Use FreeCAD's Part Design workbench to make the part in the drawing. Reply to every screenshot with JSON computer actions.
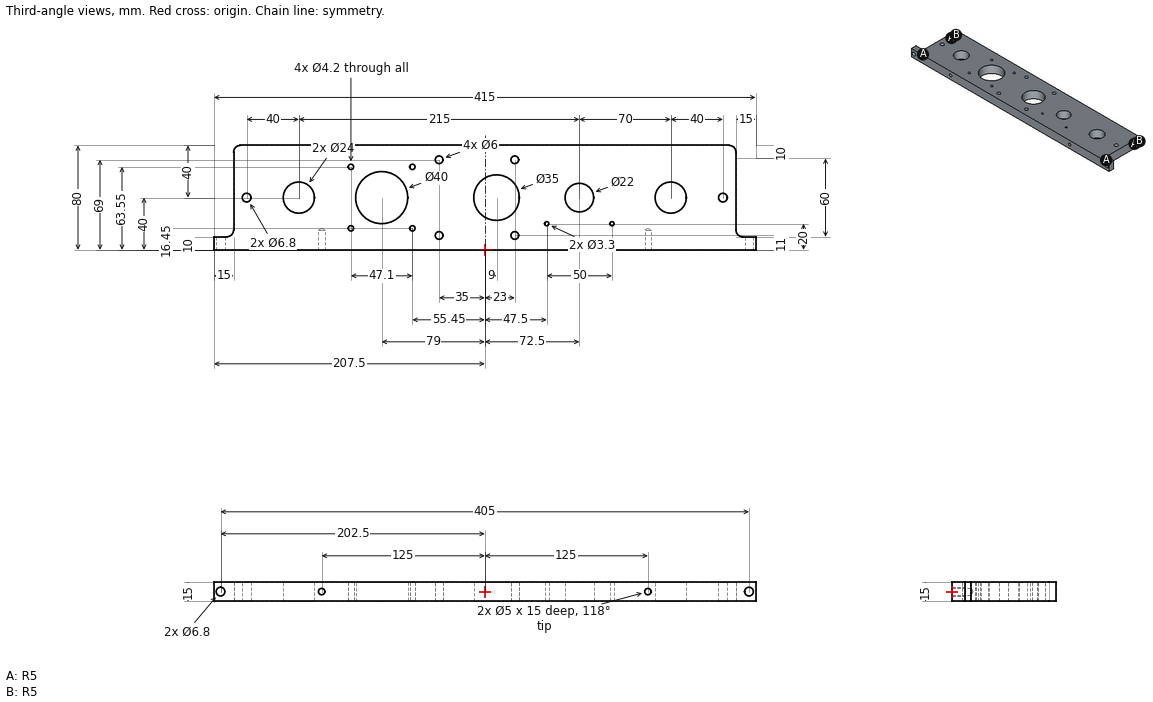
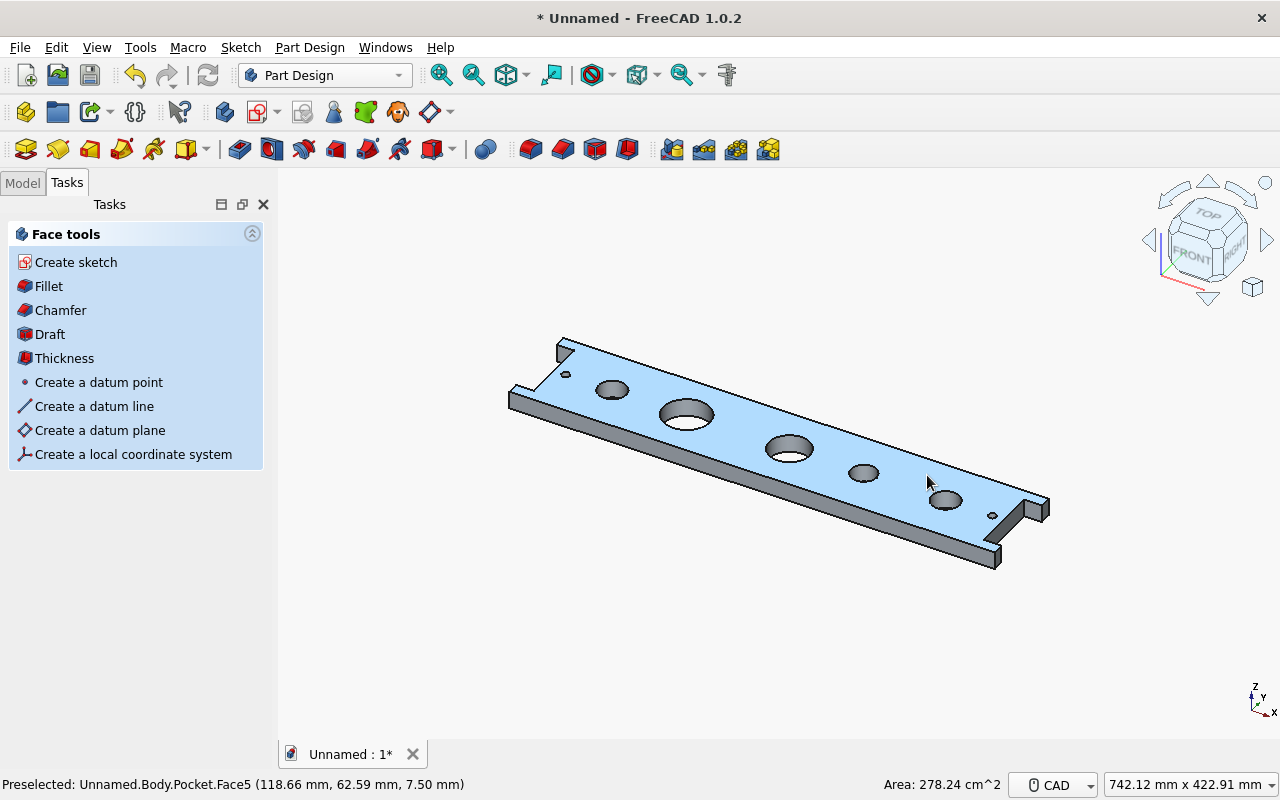
{"action": "left_click", "coordinate": [258, 112]}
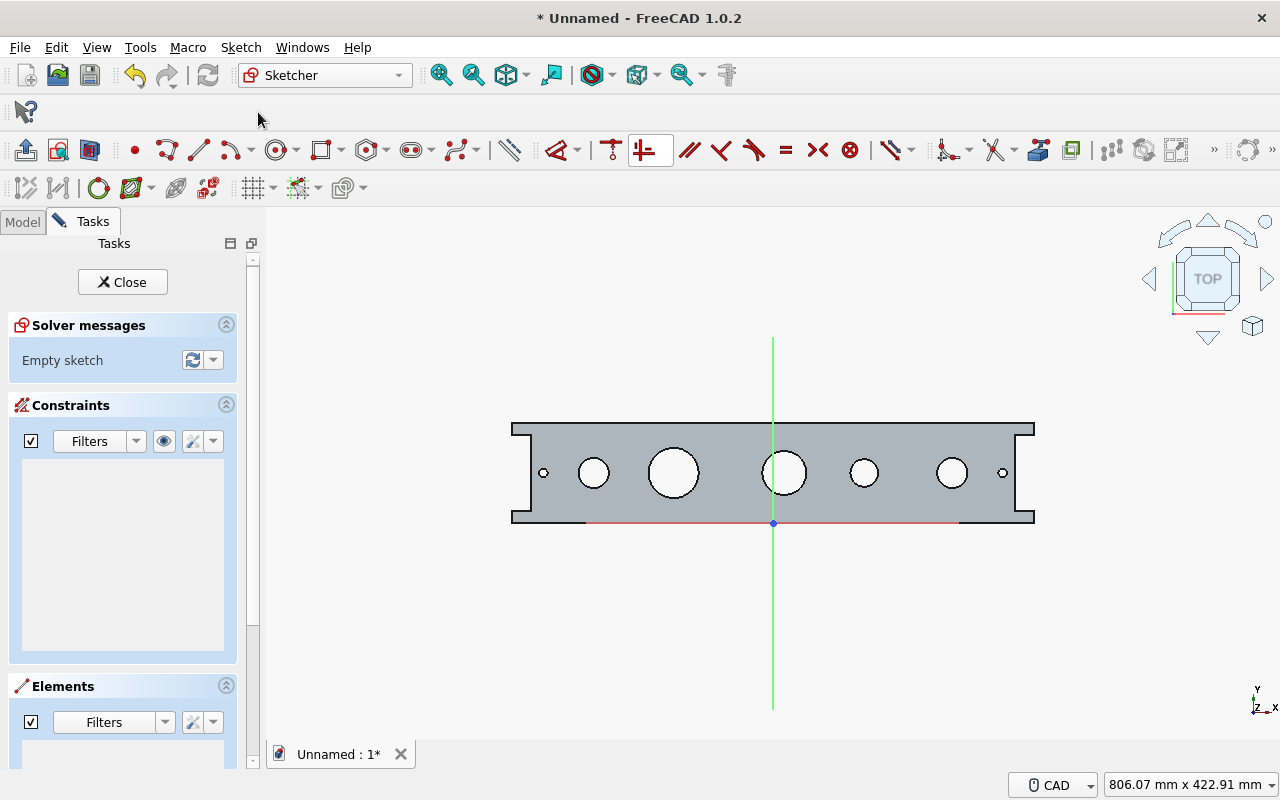
{"action": "scroll", "coordinate": [785, 480], "scroll_direction": "up", "scroll_amount": 7}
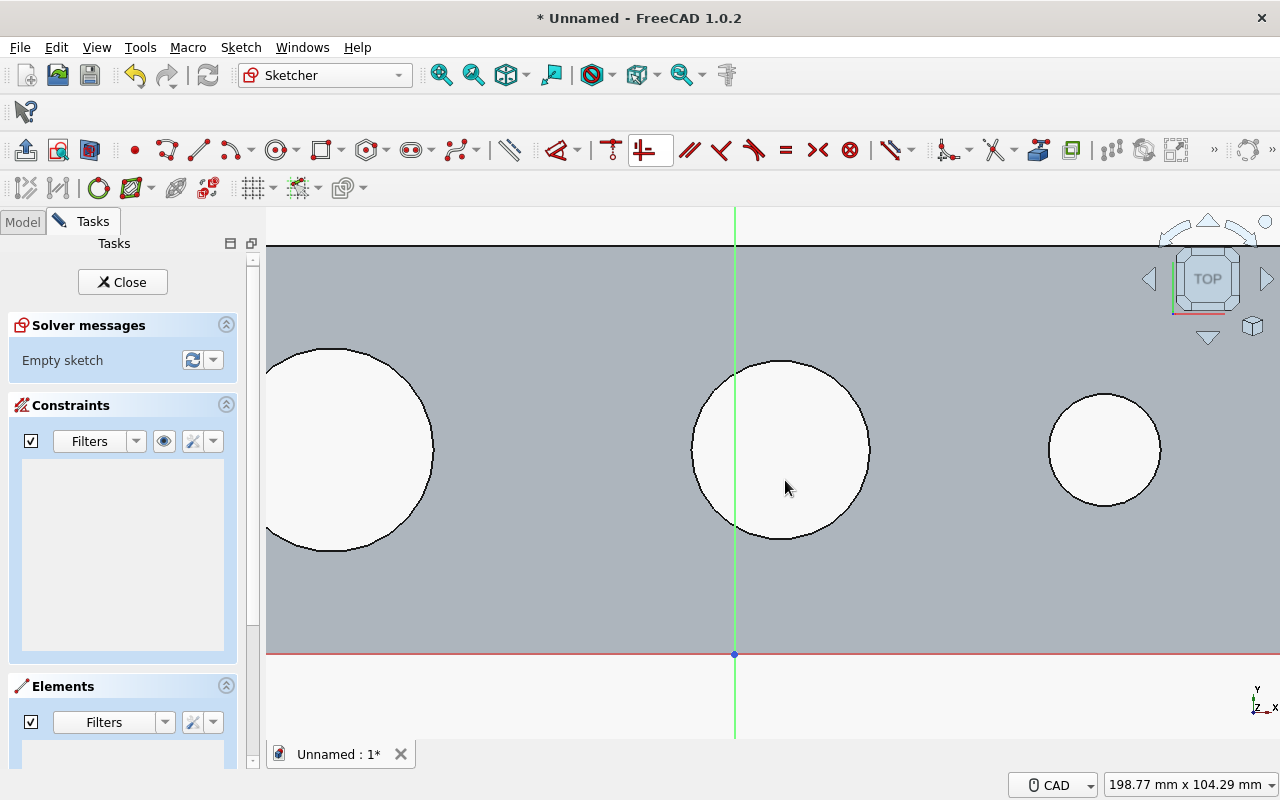
{"action": "left_click", "coordinate": [276, 150]}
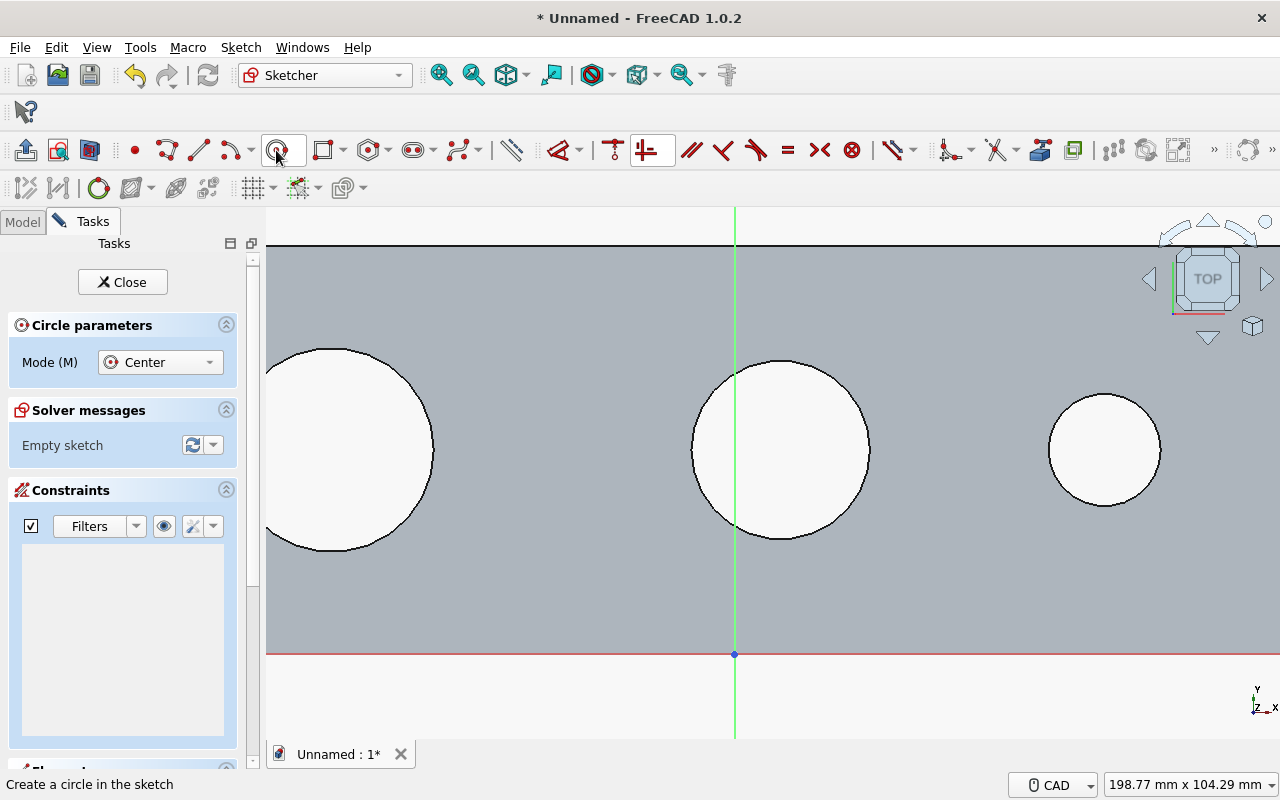
{"action": "scroll", "coordinate": [556, 302], "scroll_direction": "up", "scroll_amount": 2}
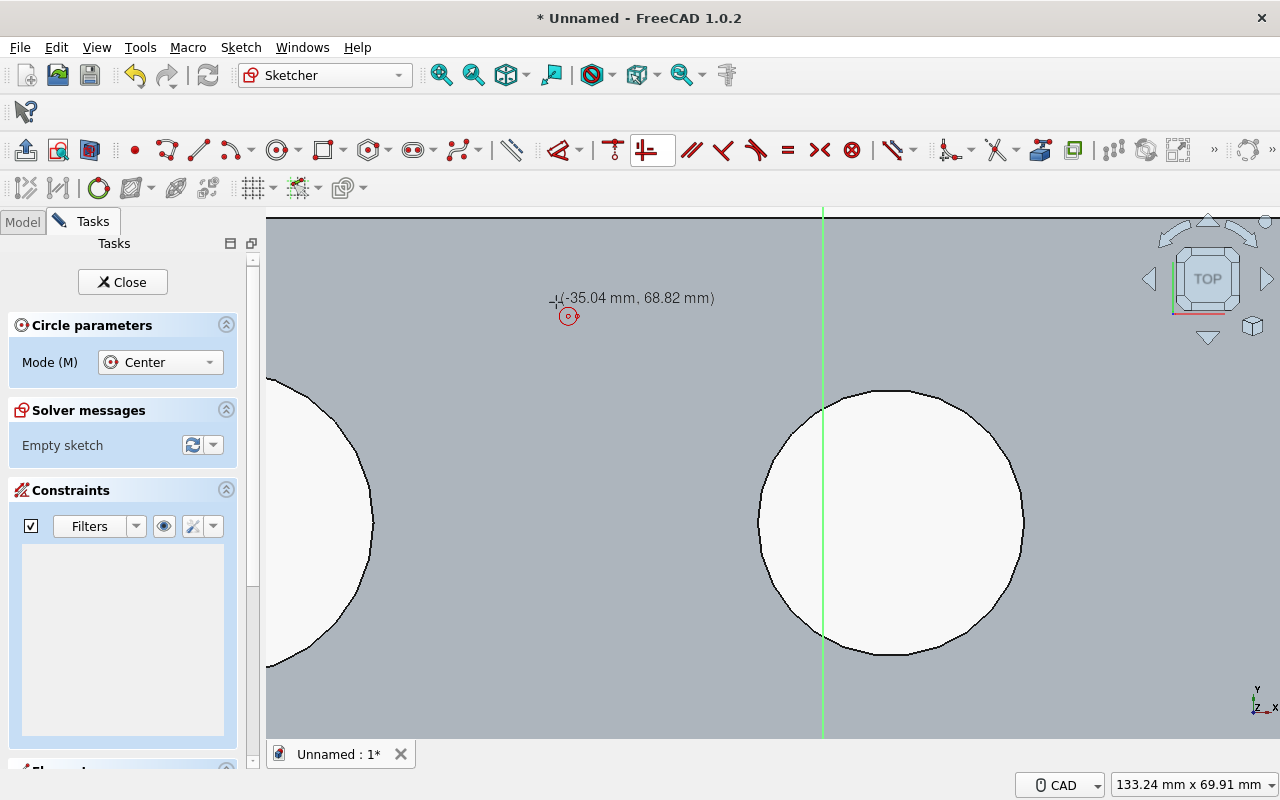
{"action": "left_click", "coordinate": [556, 302]}
{"action": "left_click", "coordinate": [572, 286]}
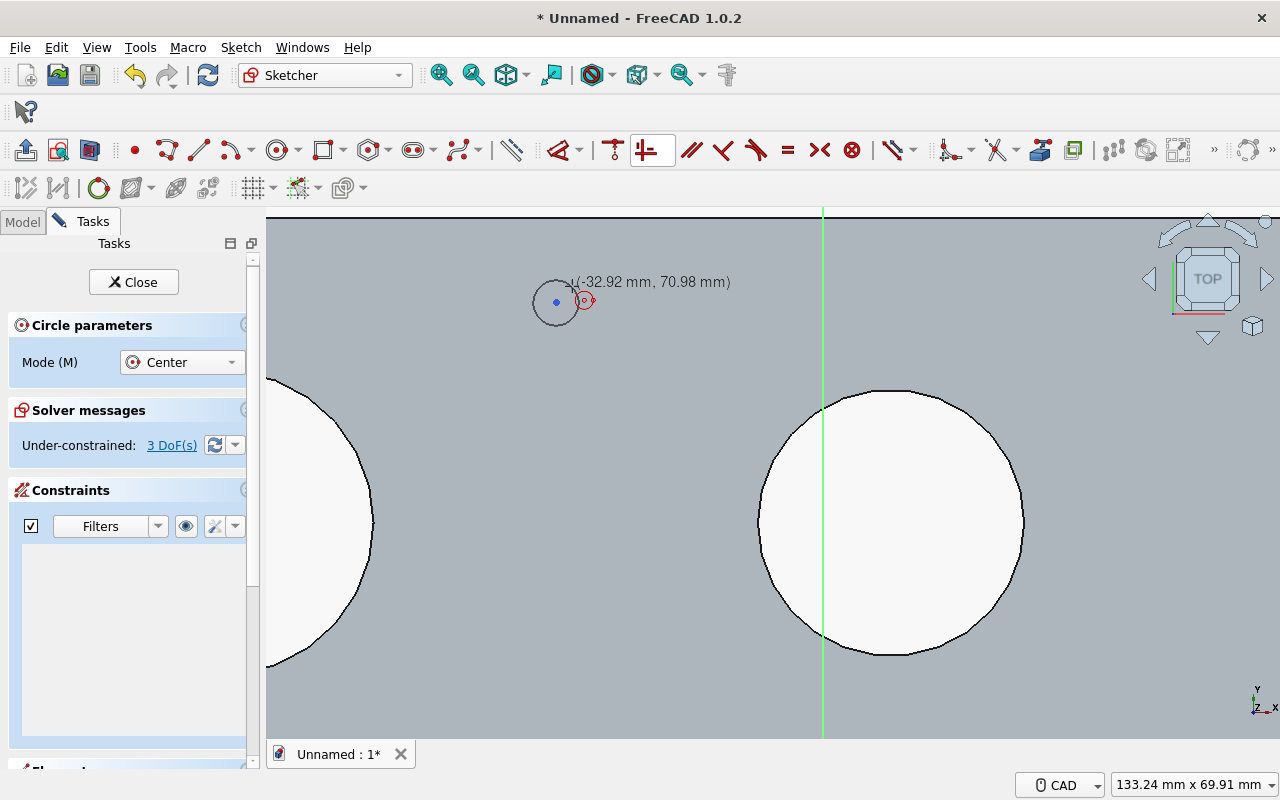
{"action": "left_click", "coordinate": [998, 302]}
{"action": "left_click", "coordinate": [1014, 286]}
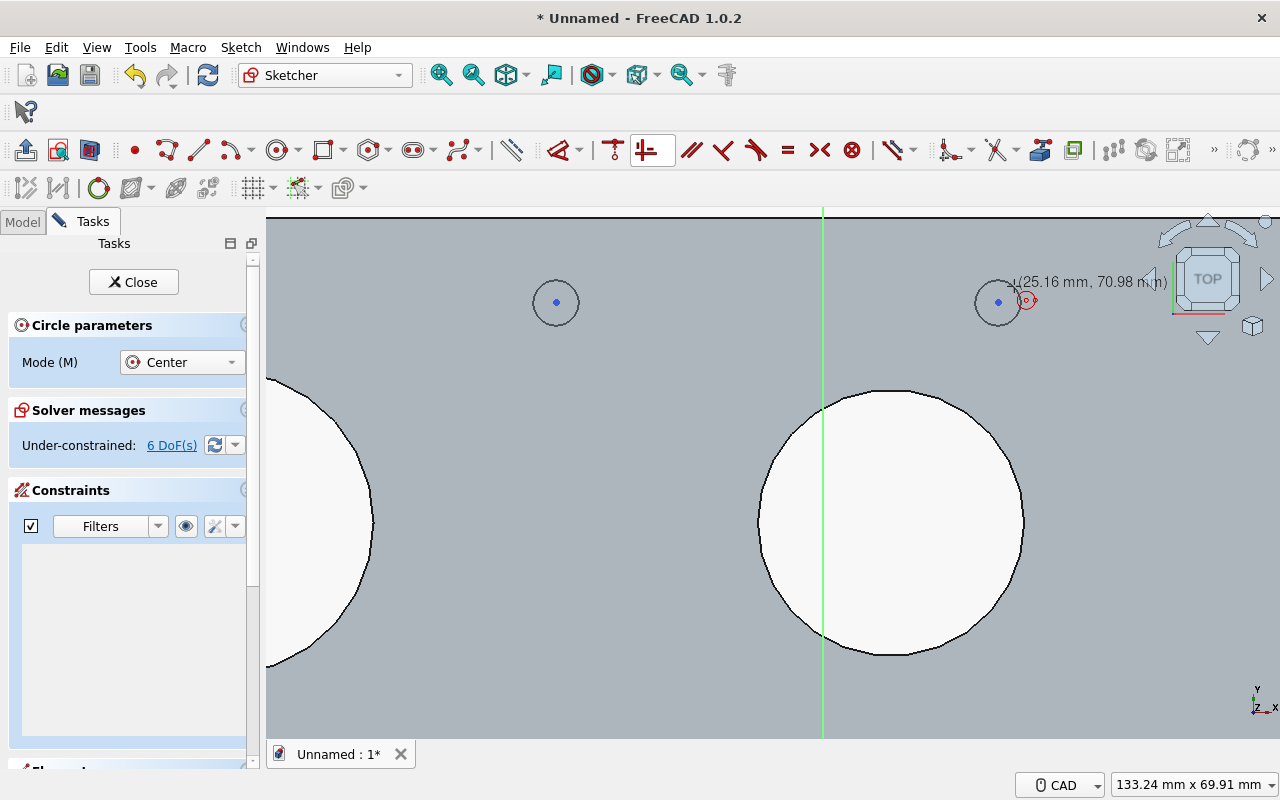
{"action": "scroll", "coordinate": [557, 310], "scroll_direction": "down", "scroll_amount": 2}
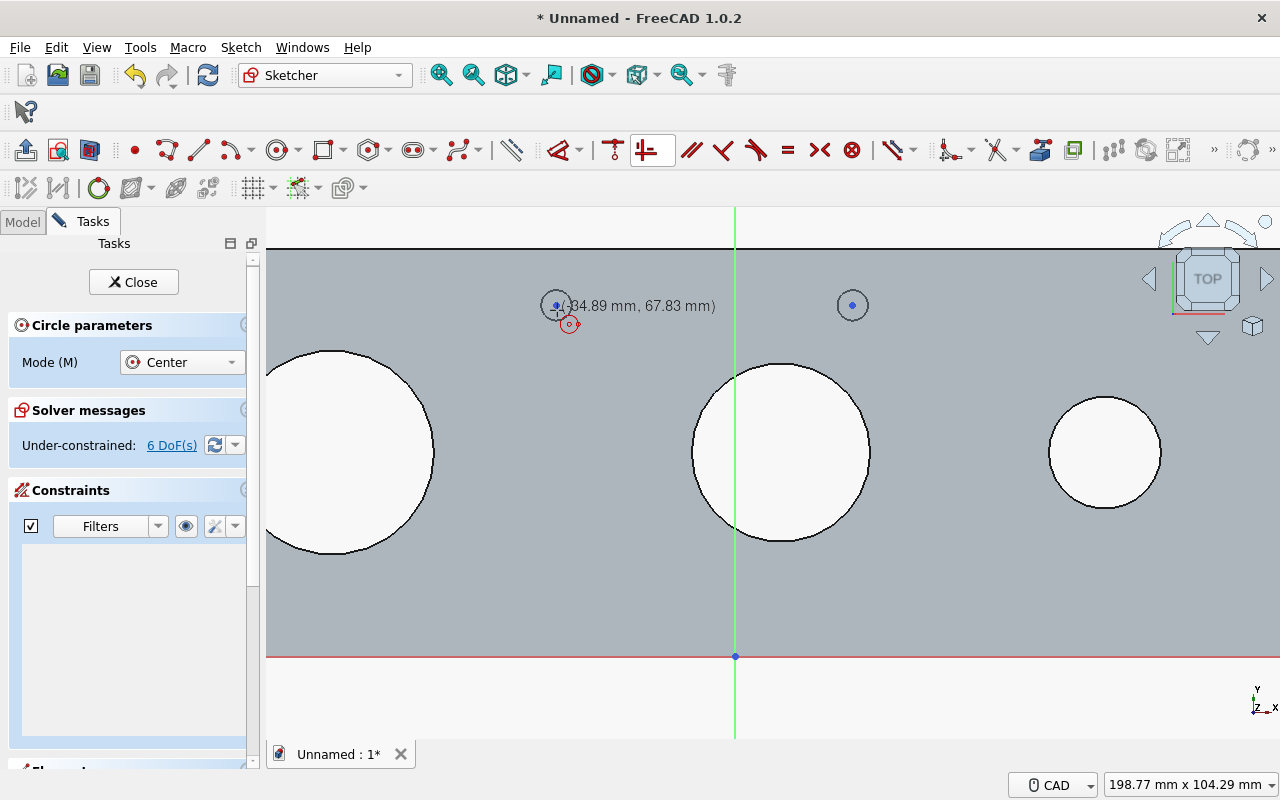
{"action": "scroll", "coordinate": [852, 601], "scroll_direction": "up", "scroll_amount": 2}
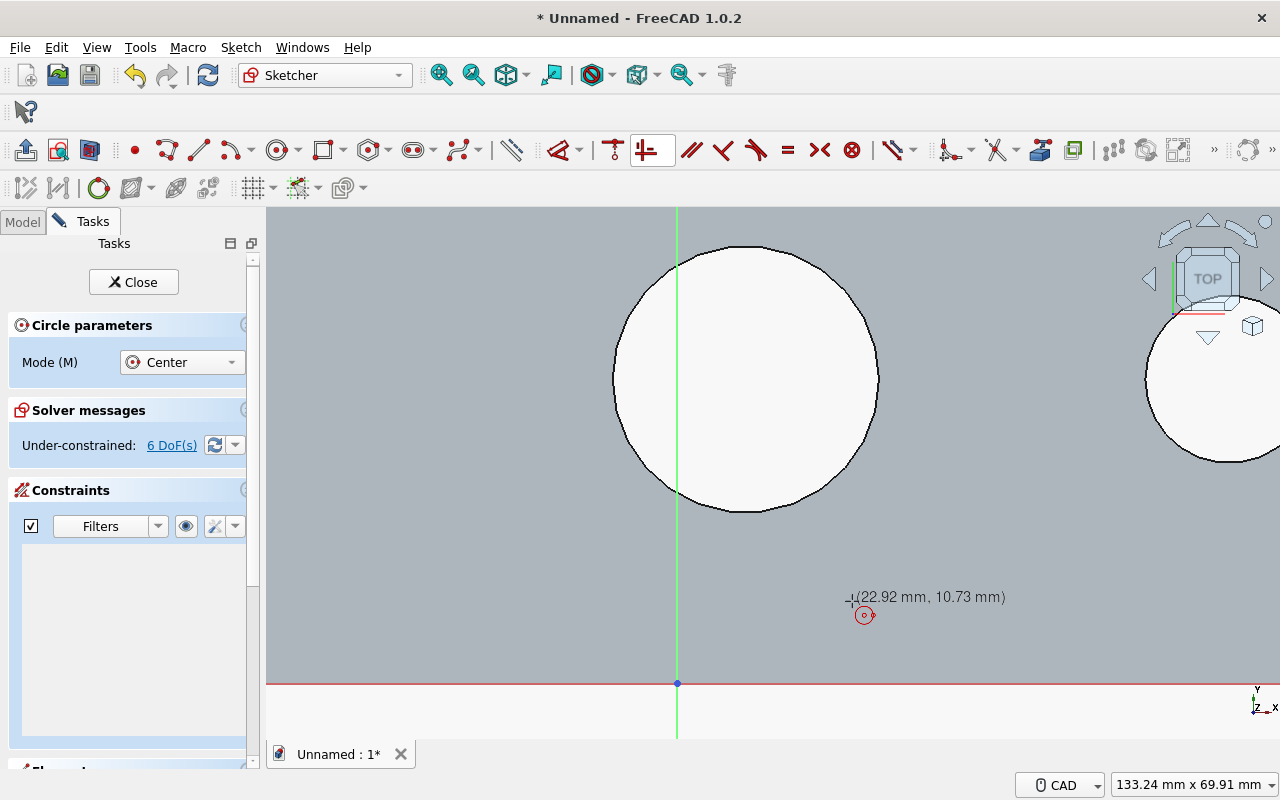
{"action": "left_click", "coordinate": [852, 600]}
{"action": "left_click", "coordinate": [869, 584]}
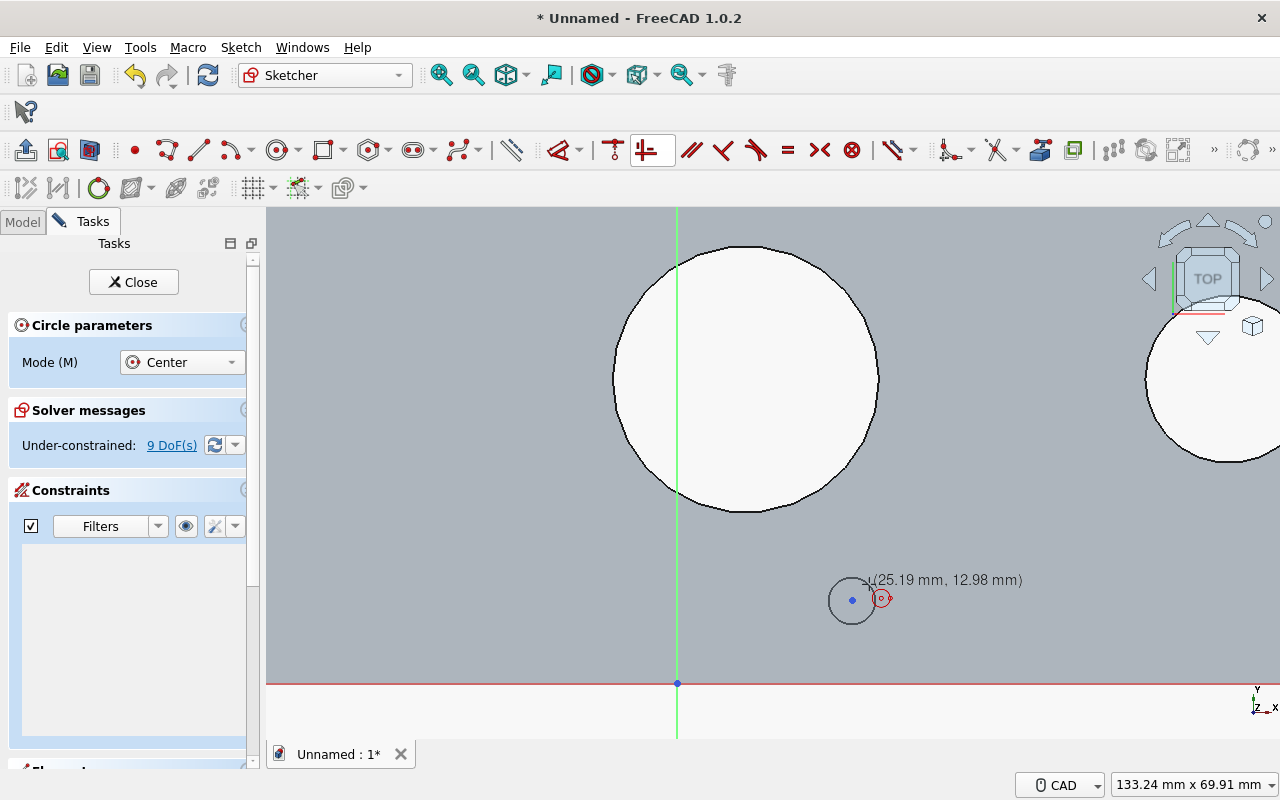
{"action": "left_click", "coordinate": [411, 600]}
{"action": "left_click", "coordinate": [427, 584]}
{"action": "key", "text": "Escape"}